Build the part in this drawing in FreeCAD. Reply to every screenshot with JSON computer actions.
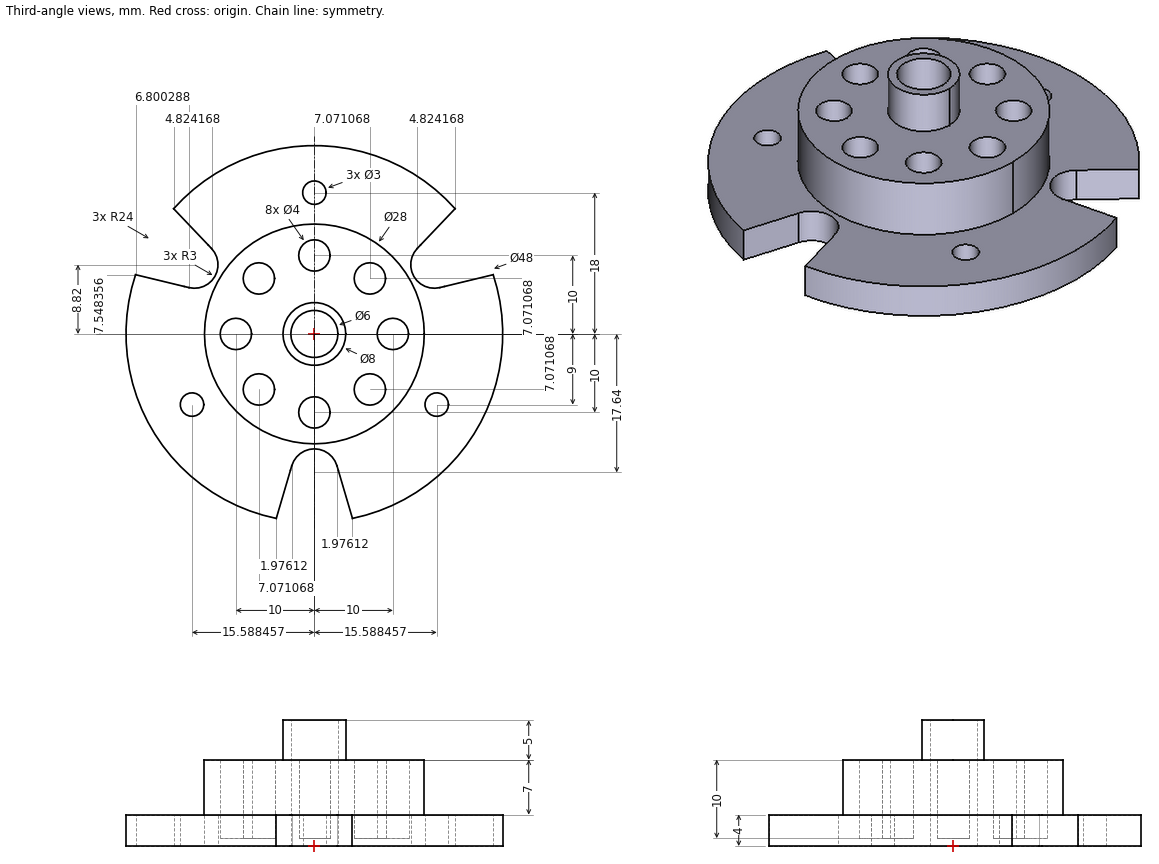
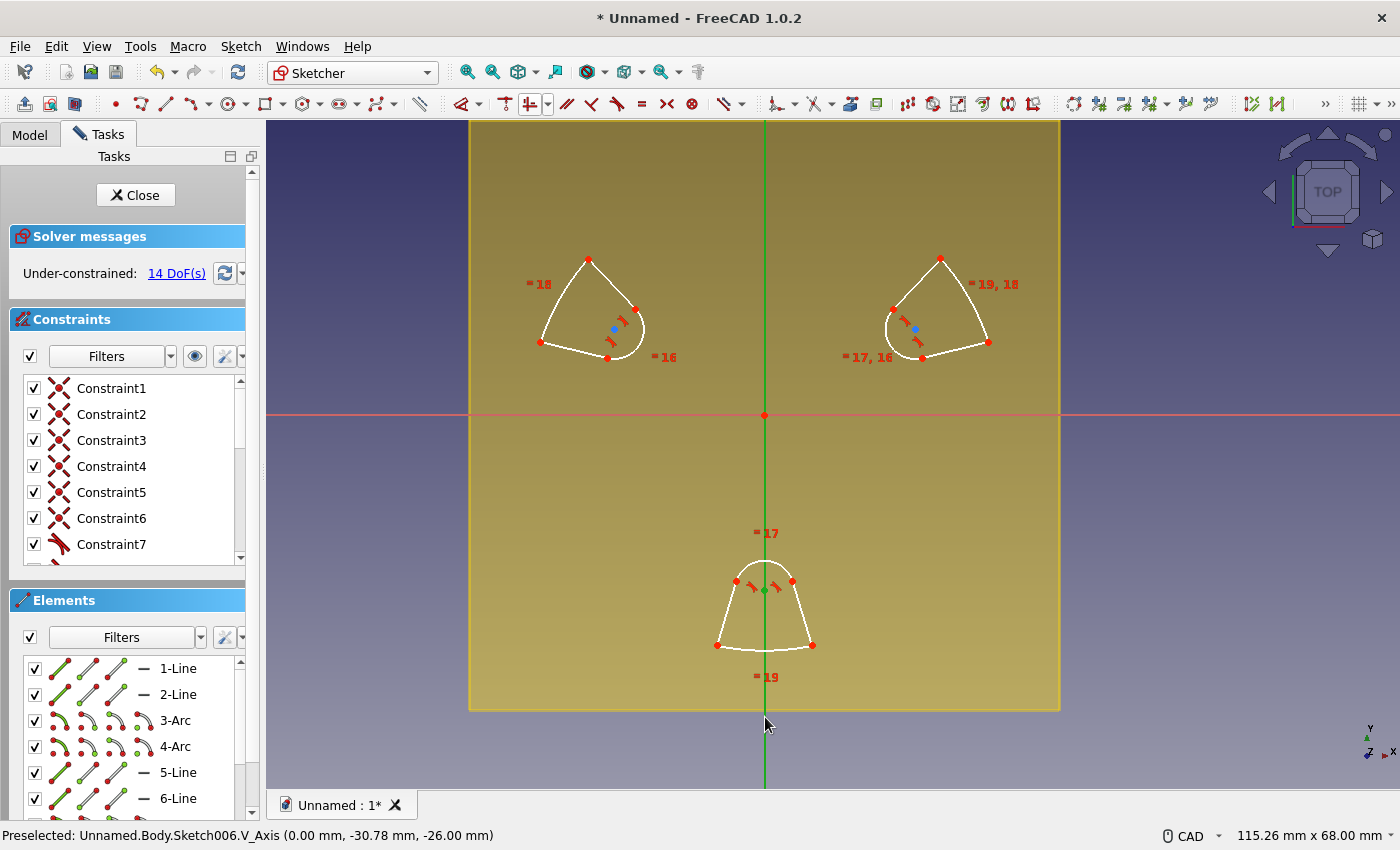
{"action": "key", "text": "c"}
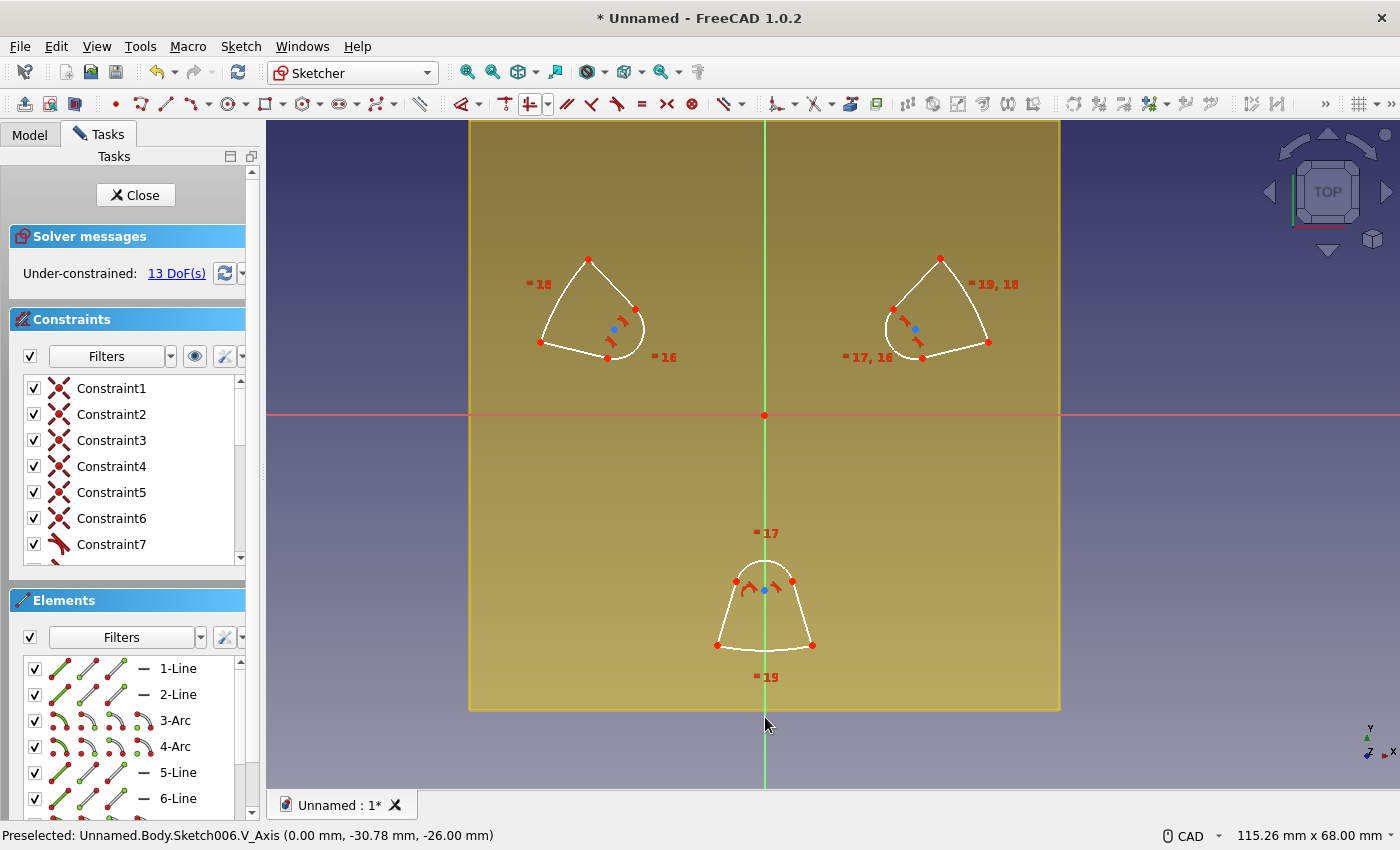
{"action": "left_click", "coordinate": [614, 329]}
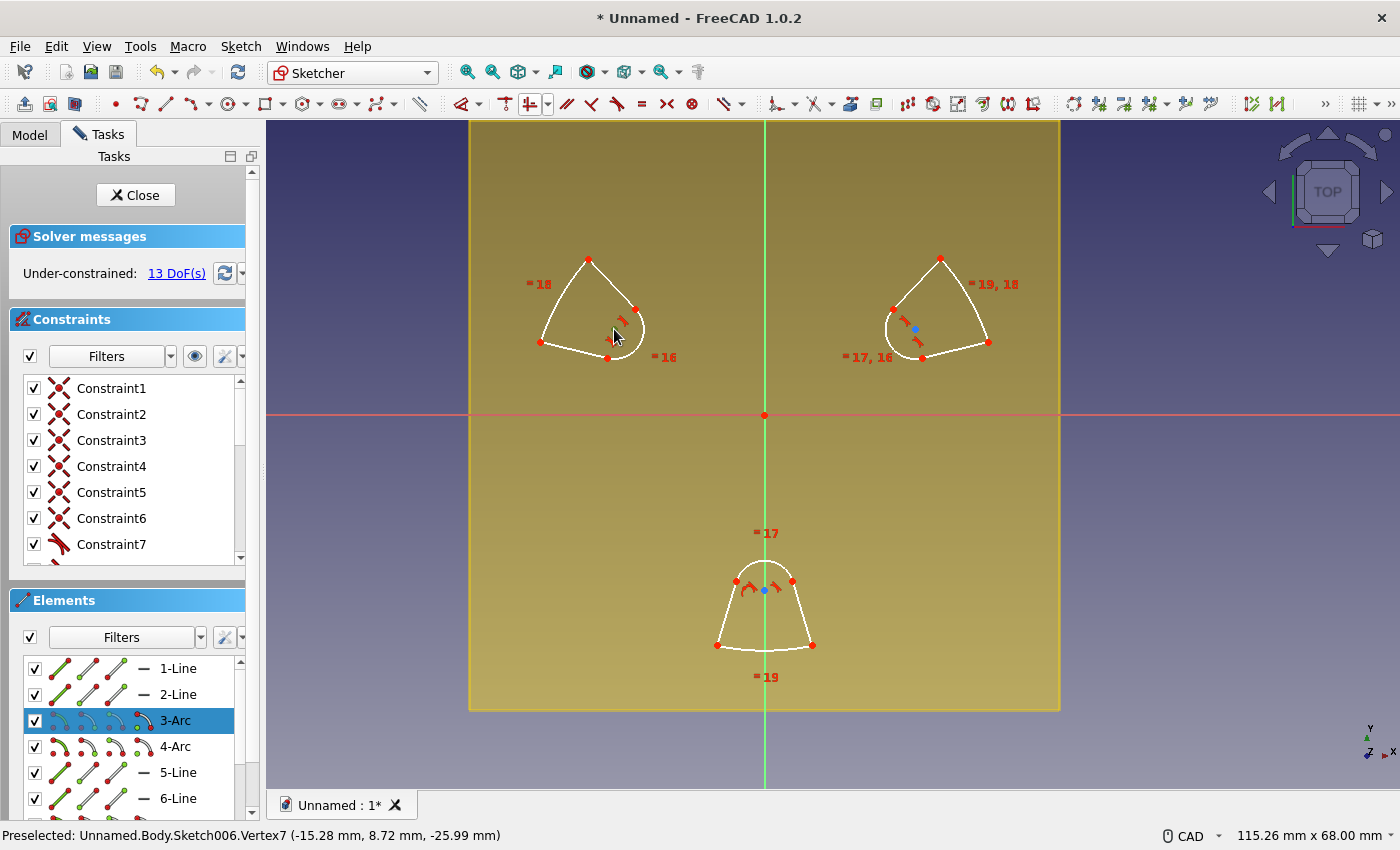
{"action": "left_click", "coordinate": [915, 329]}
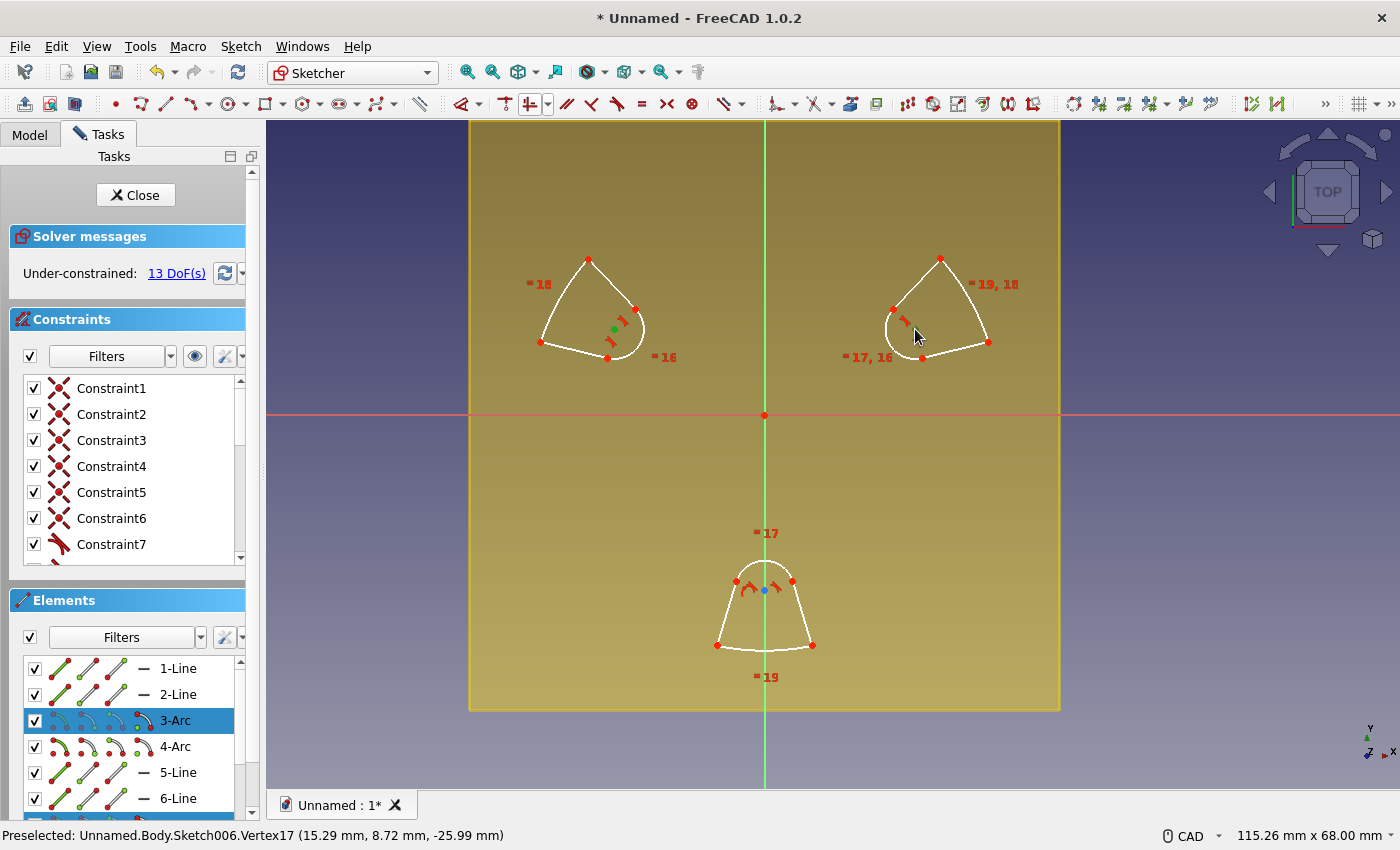
{"action": "left_click", "coordinate": [765, 717]}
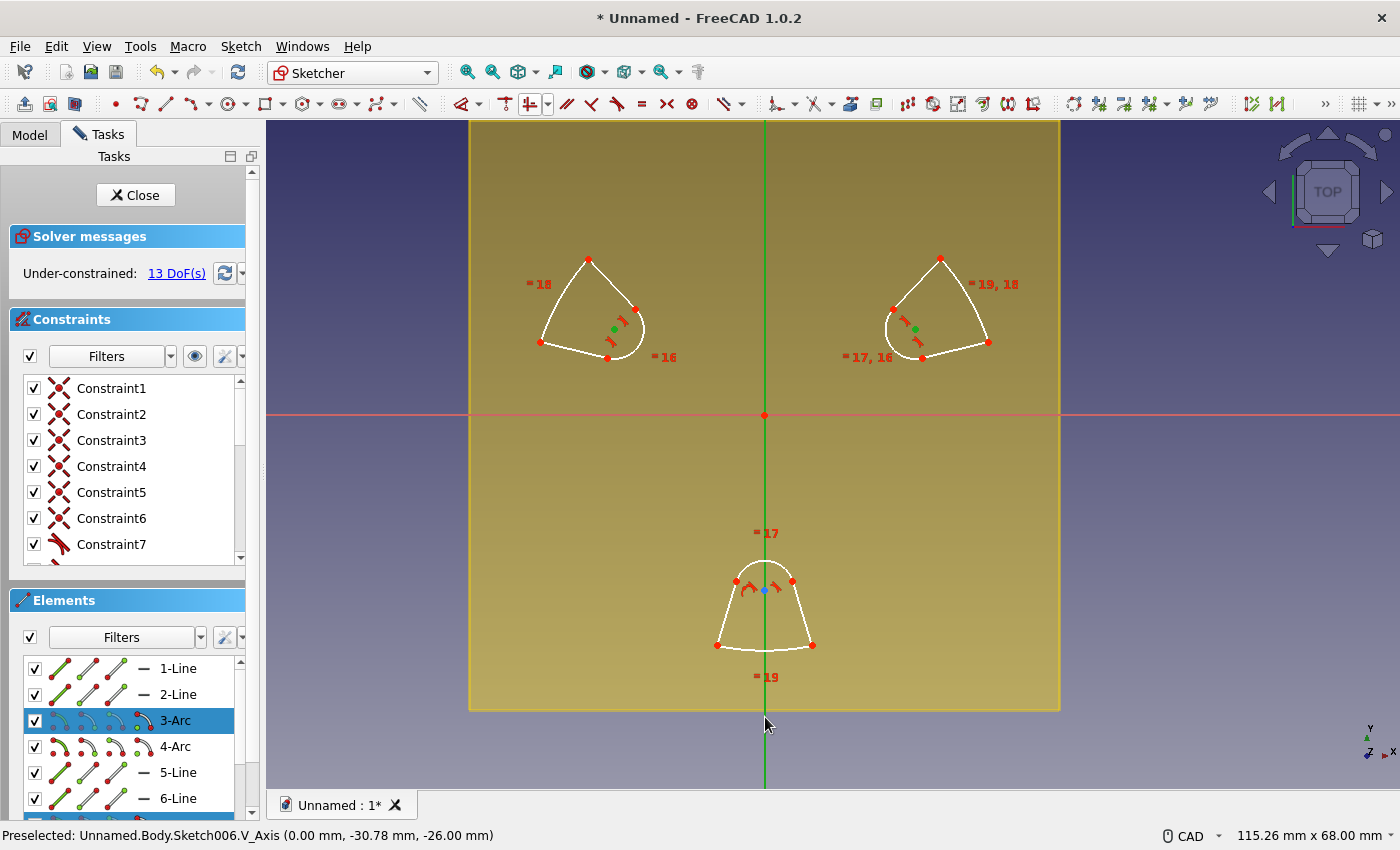
{"action": "key", "text": "s"}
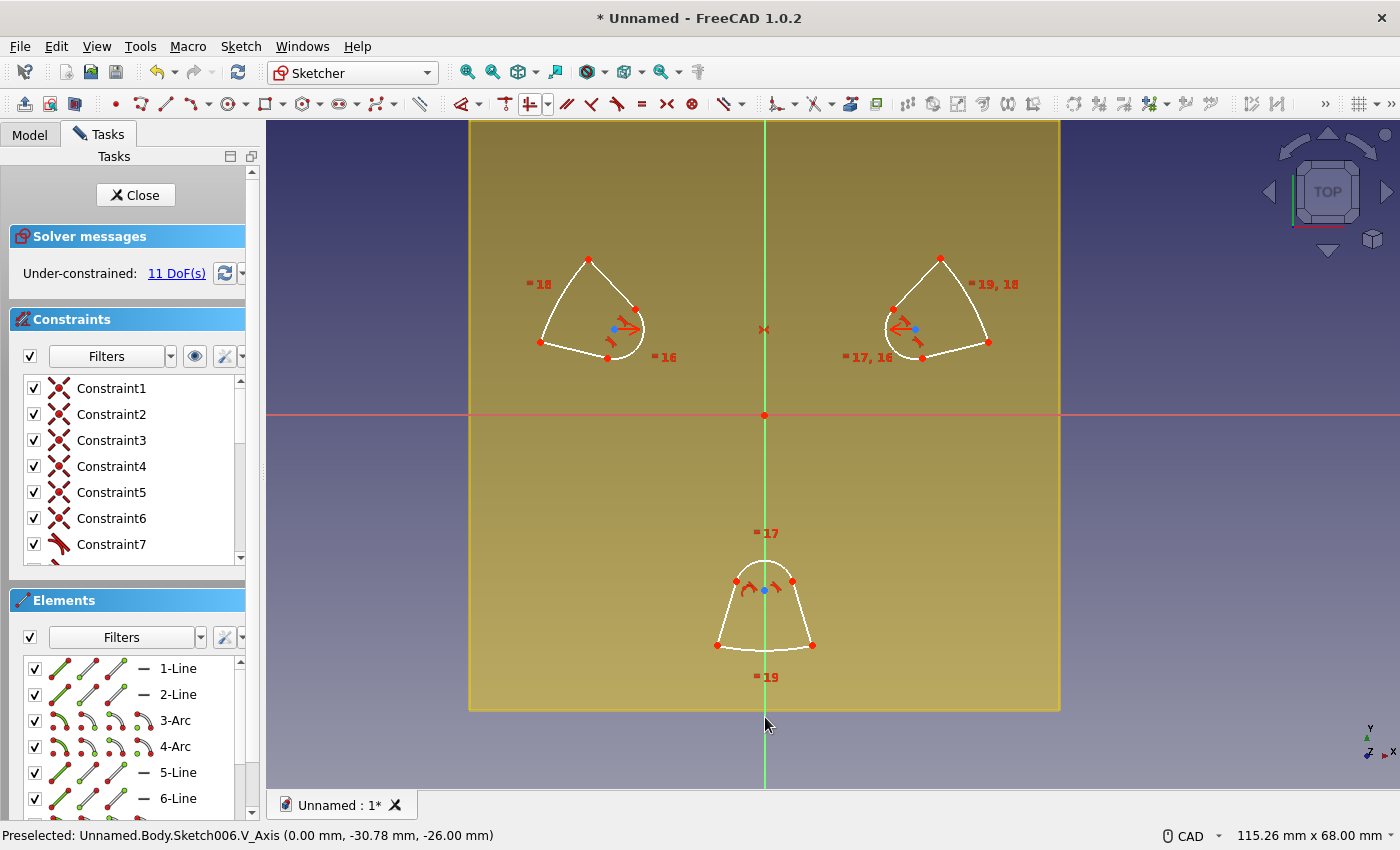
{"action": "key", "text": "d"}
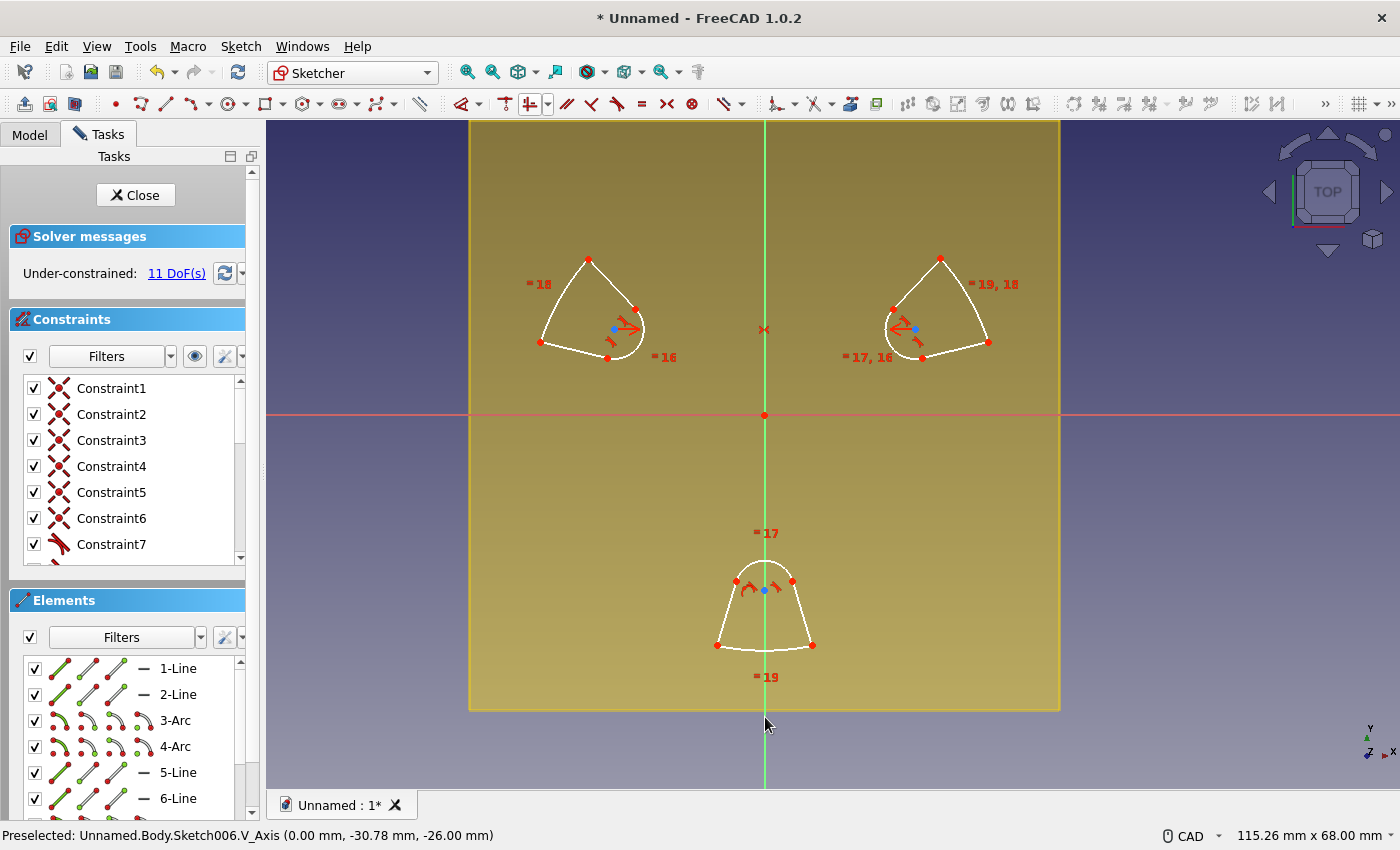
{"action": "scroll", "coordinate": [629, 355], "scroll_direction": "up", "scroll_amount": 2}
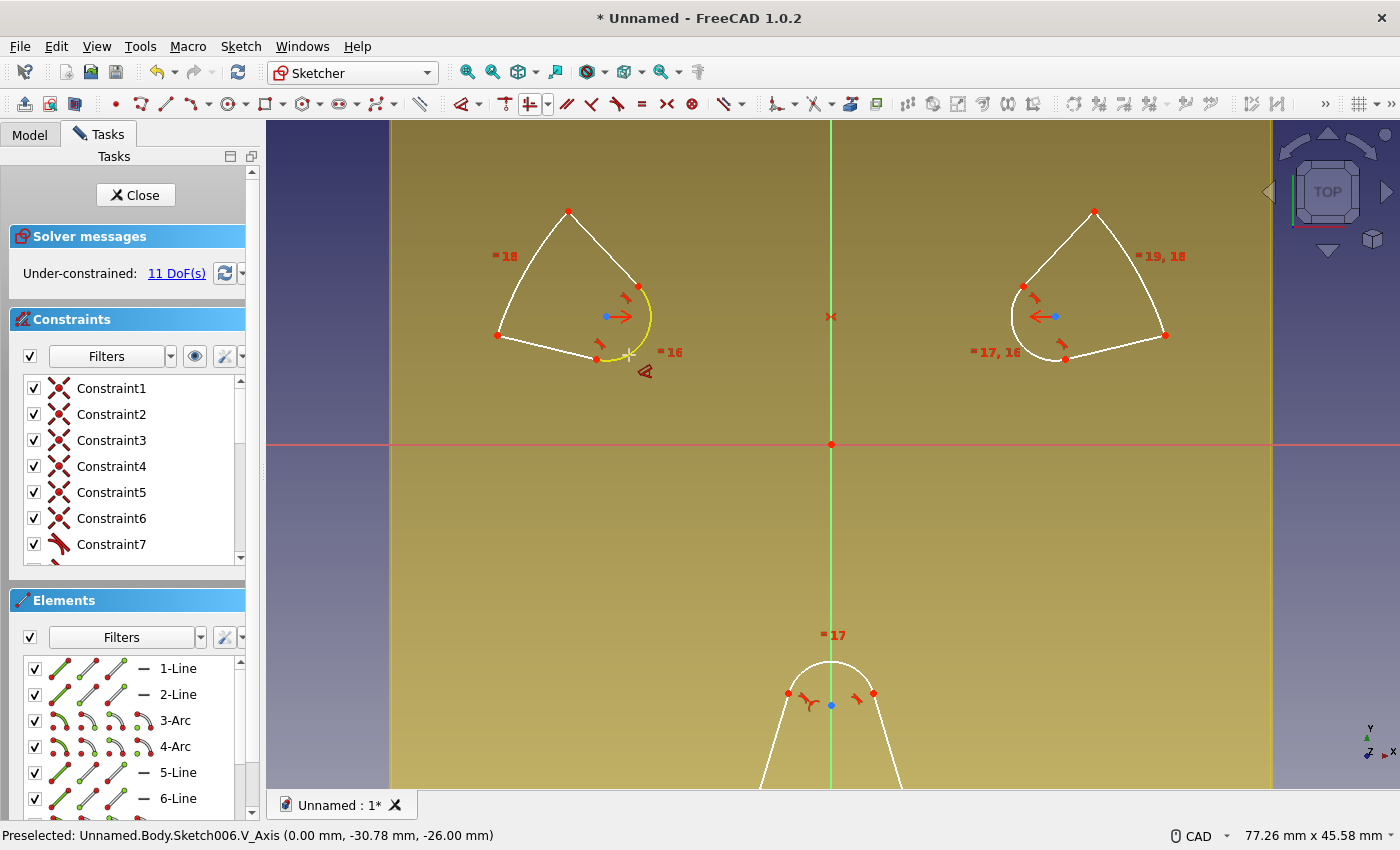
{"action": "left_click", "coordinate": [629, 355]}
{"action": "left_click", "coordinate": [645, 383]}